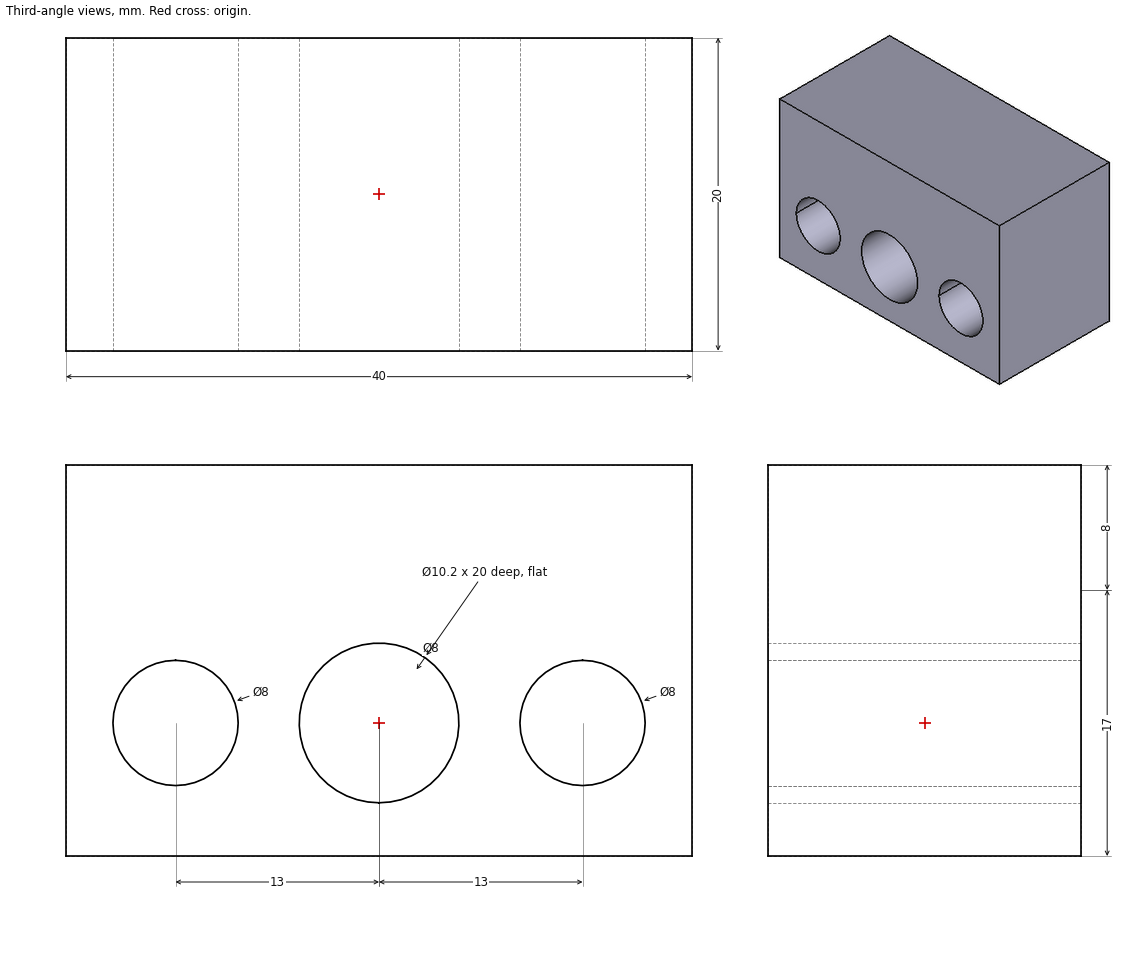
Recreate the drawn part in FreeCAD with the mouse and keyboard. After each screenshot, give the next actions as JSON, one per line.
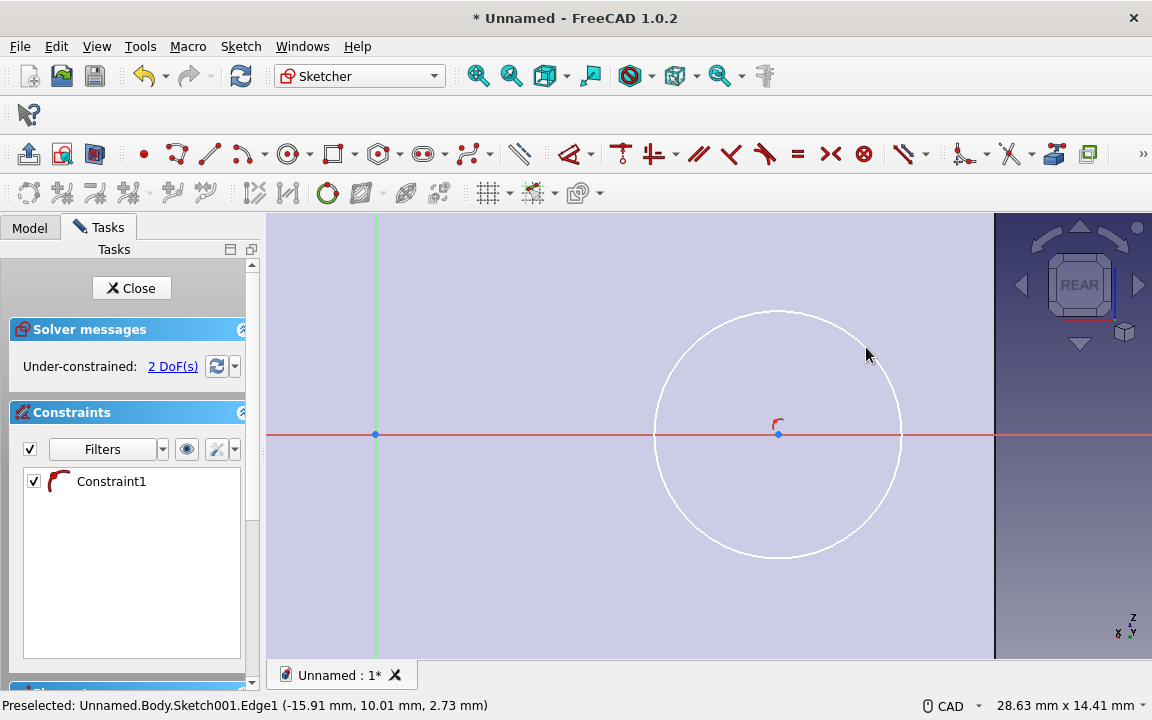
{"action": "left_click", "coordinate": [568, 154]}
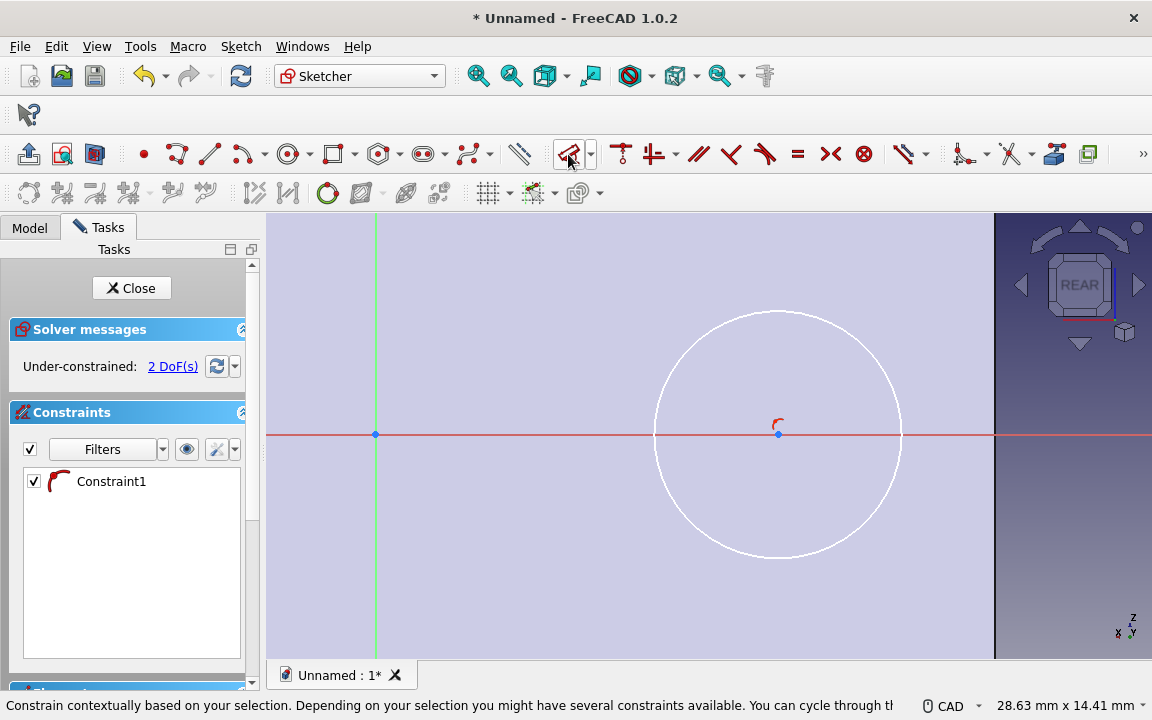
{"action": "left_click", "coordinate": [865, 347]}
{"action": "left_click", "coordinate": [888, 324]}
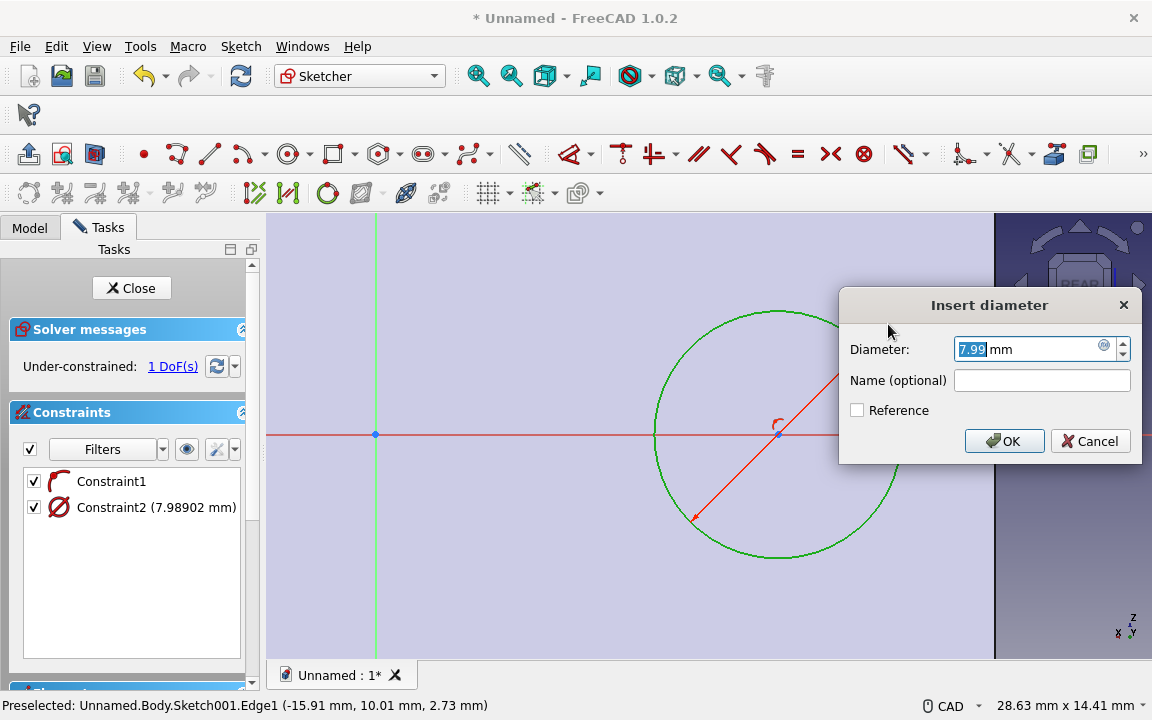
{"action": "type", "text": "8"}
{"action": "key", "text": "Return"}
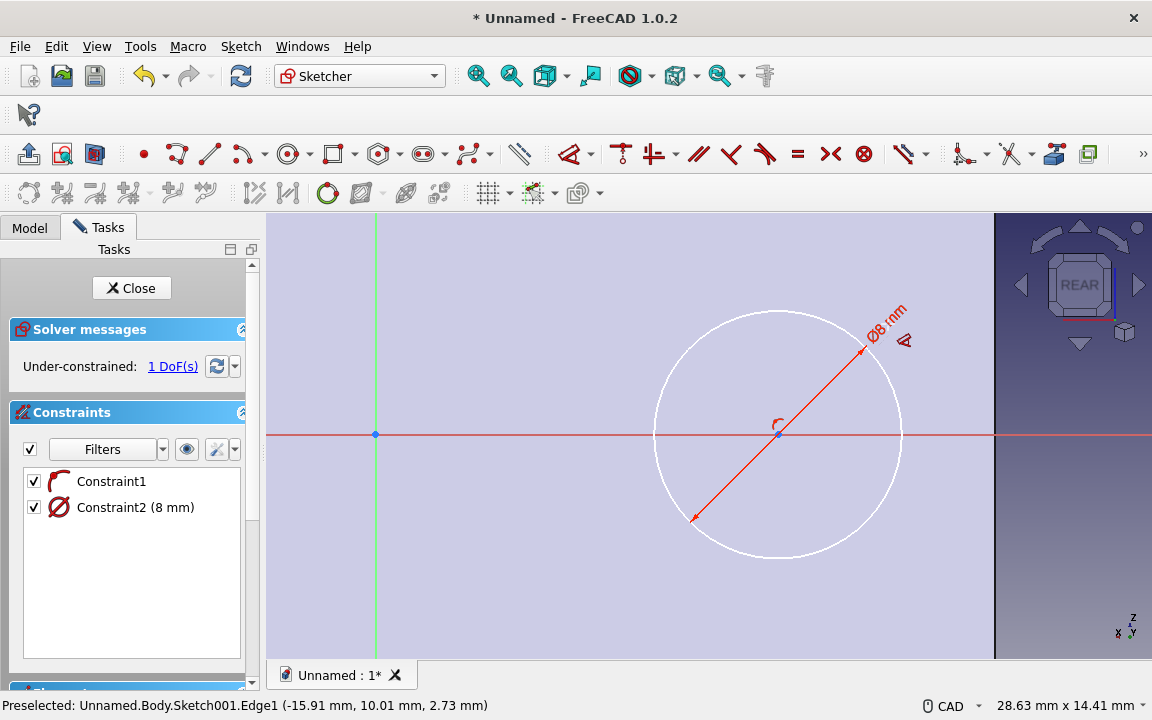
{"action": "left_click", "coordinate": [778, 435]}
{"action": "left_click", "coordinate": [577, 469]}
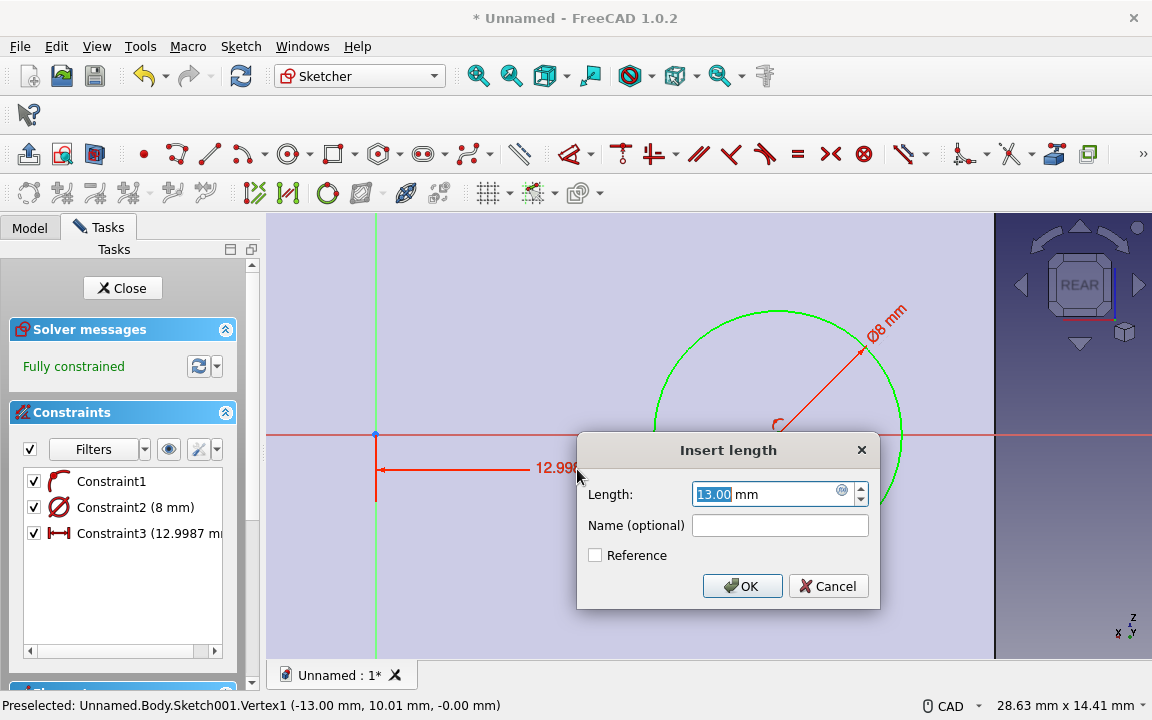
{"action": "type", "text": "13"}
{"action": "key", "text": "Return"}
{"action": "key", "text": "Escape"}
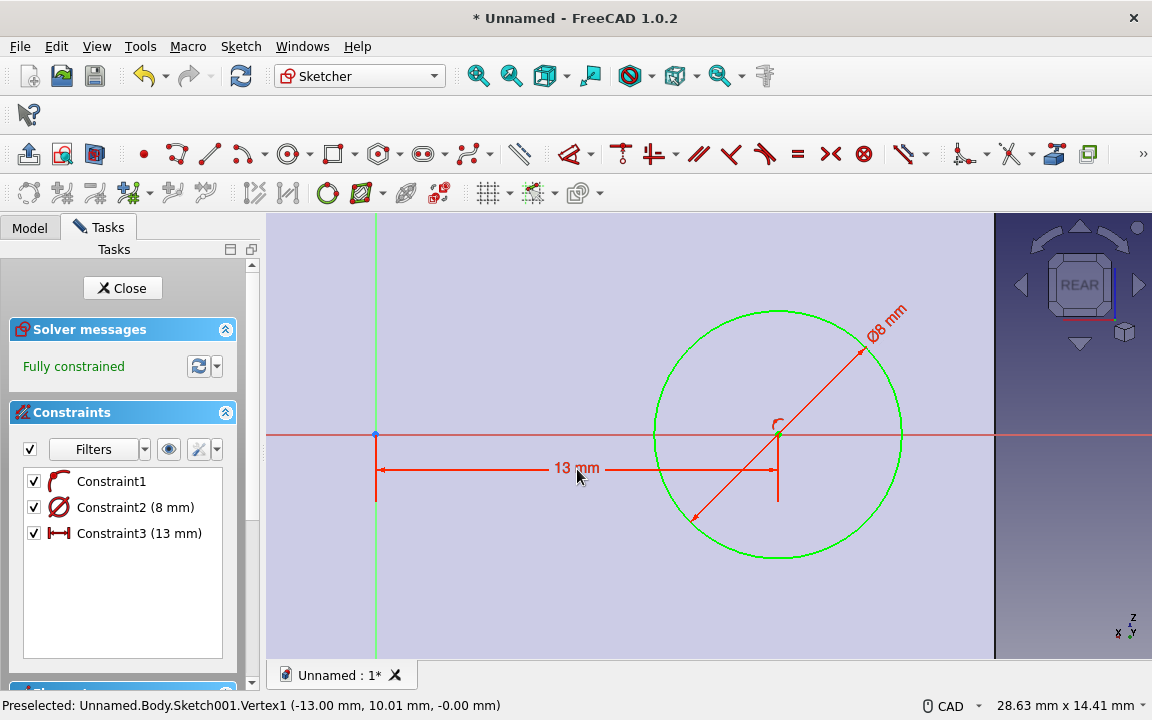
{"action": "left_click", "coordinate": [123, 288]}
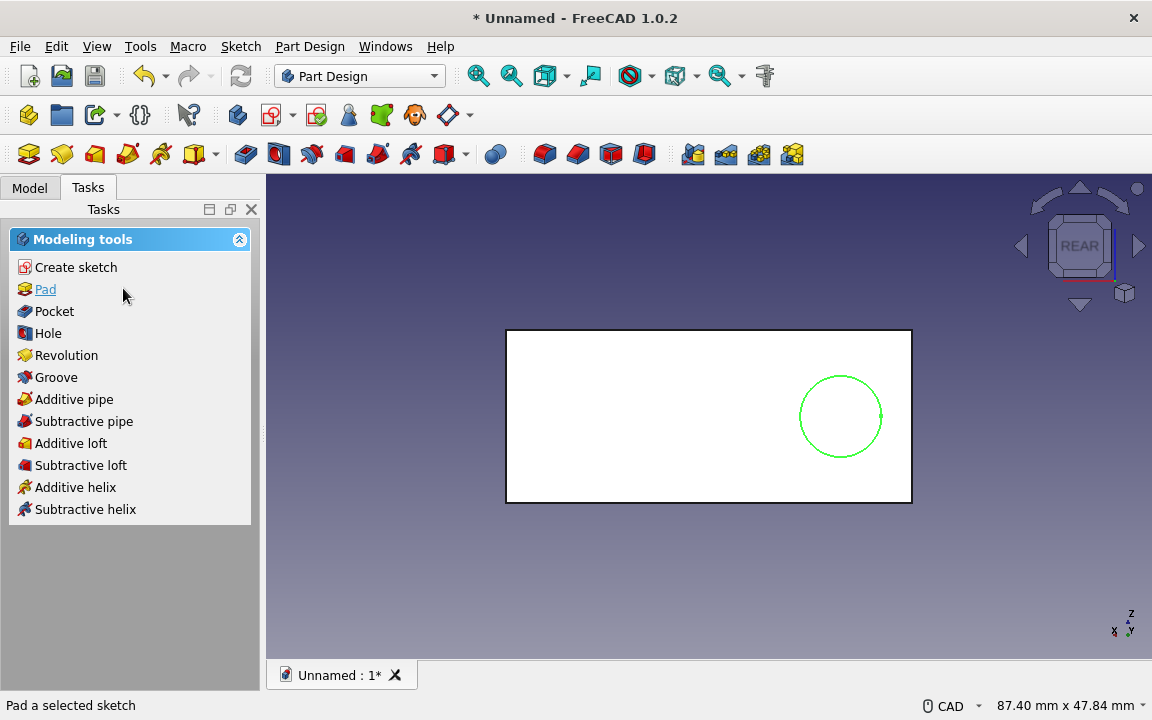
{"action": "left_click", "coordinate": [246, 154]}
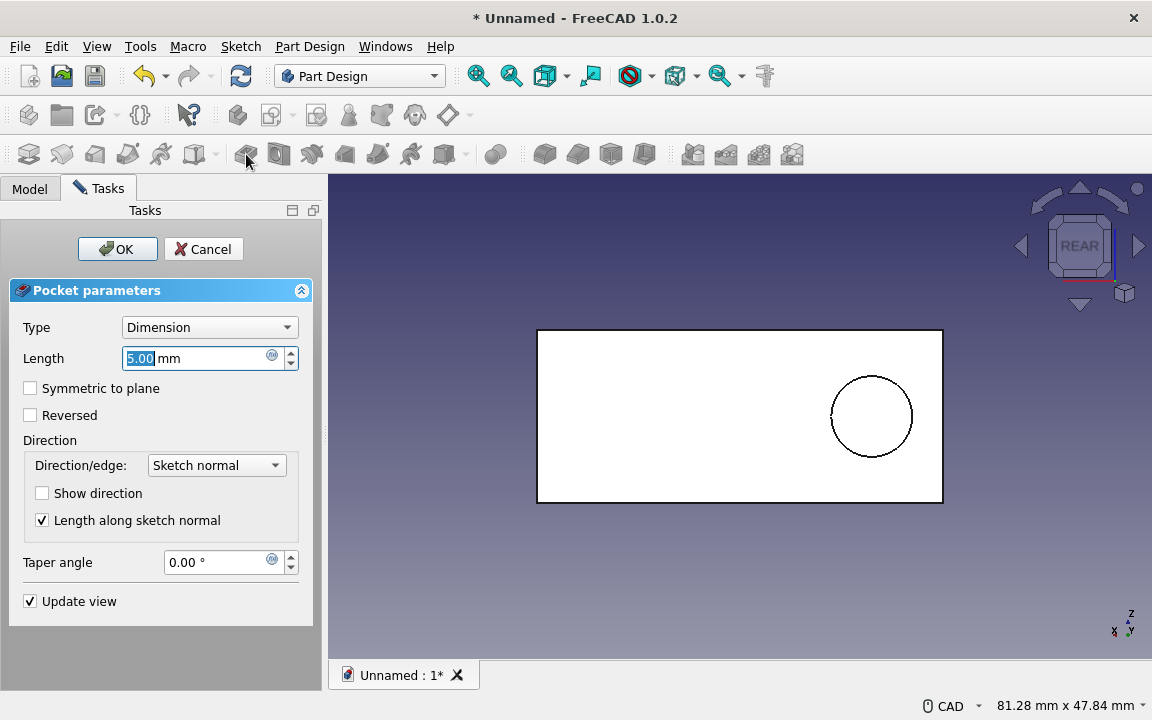
{"action": "left_click", "coordinate": [210, 328]}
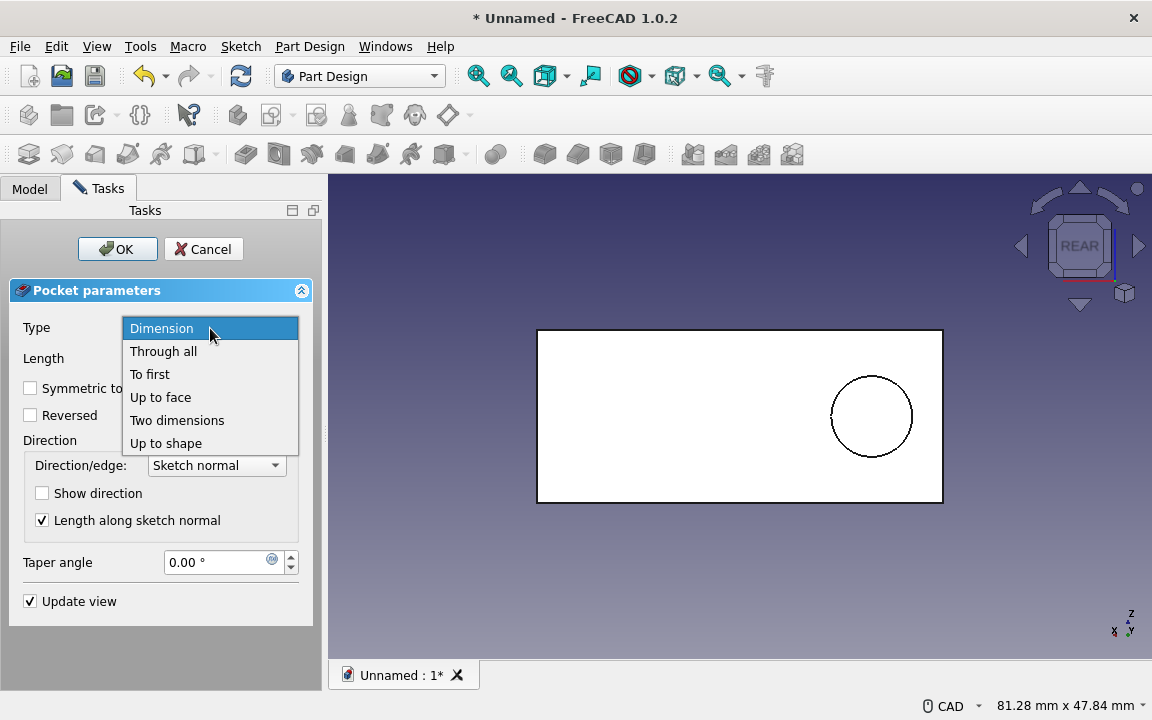
{"action": "left_click", "coordinate": [208, 374]}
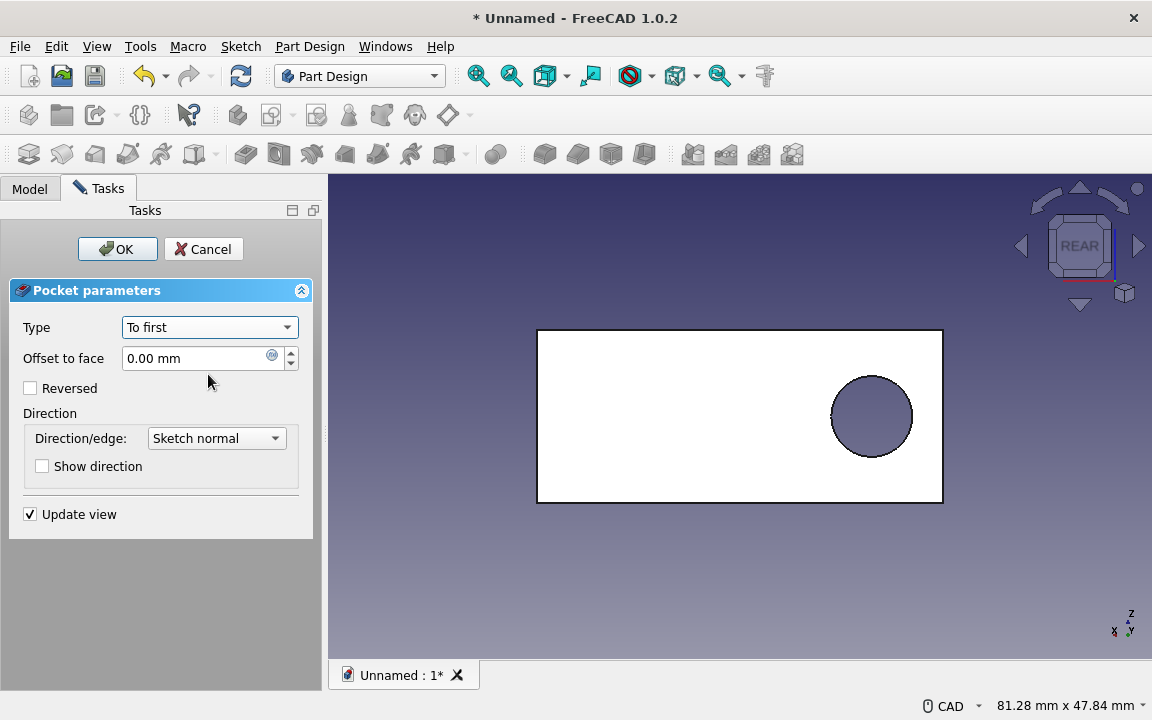
{"action": "left_click", "coordinate": [118, 249]}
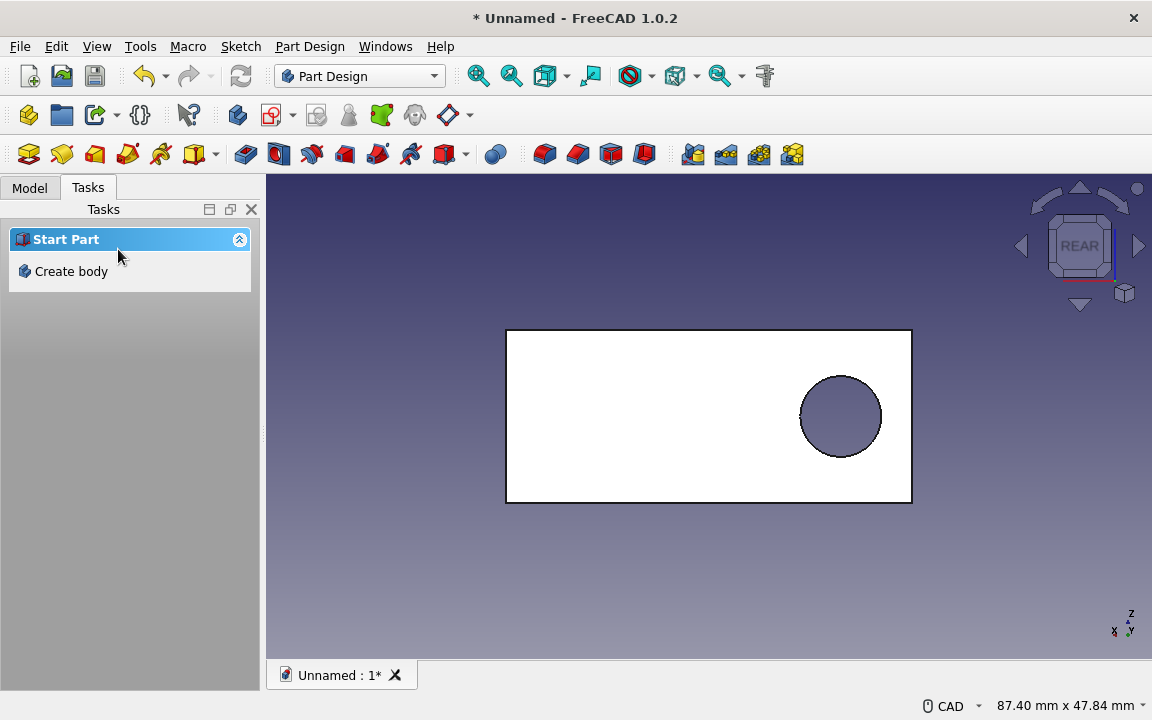
{"action": "left_click", "coordinate": [593, 415]}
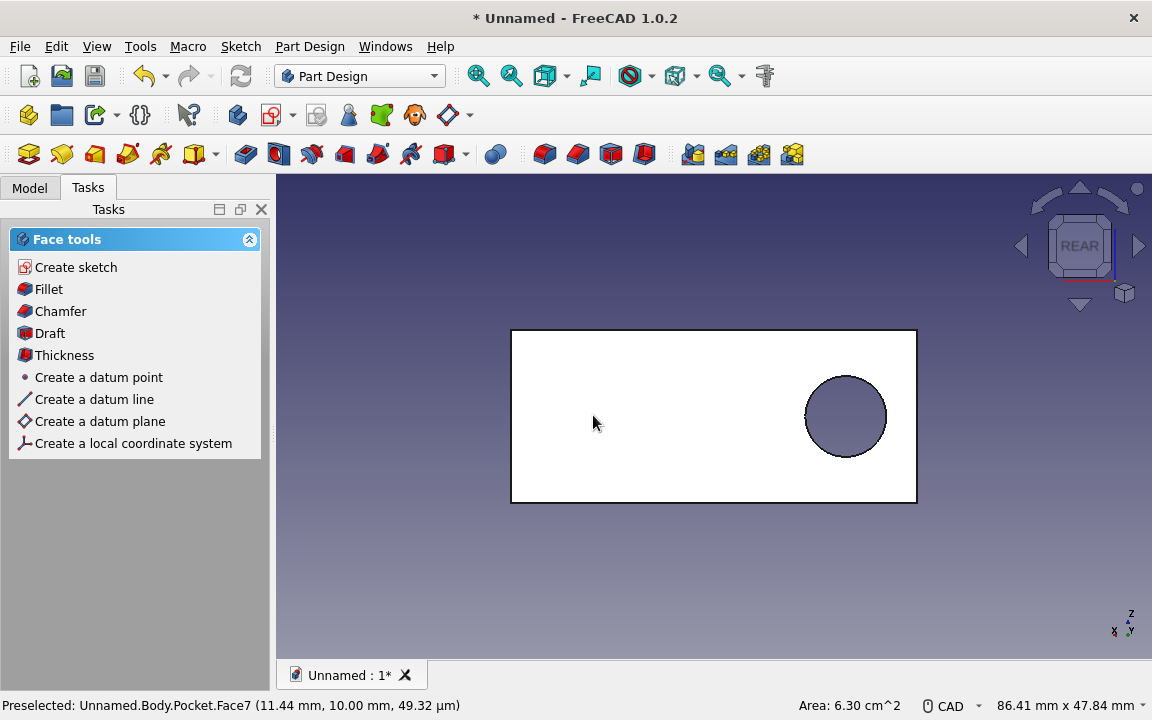
{"action": "left_click", "coordinate": [270, 116]}